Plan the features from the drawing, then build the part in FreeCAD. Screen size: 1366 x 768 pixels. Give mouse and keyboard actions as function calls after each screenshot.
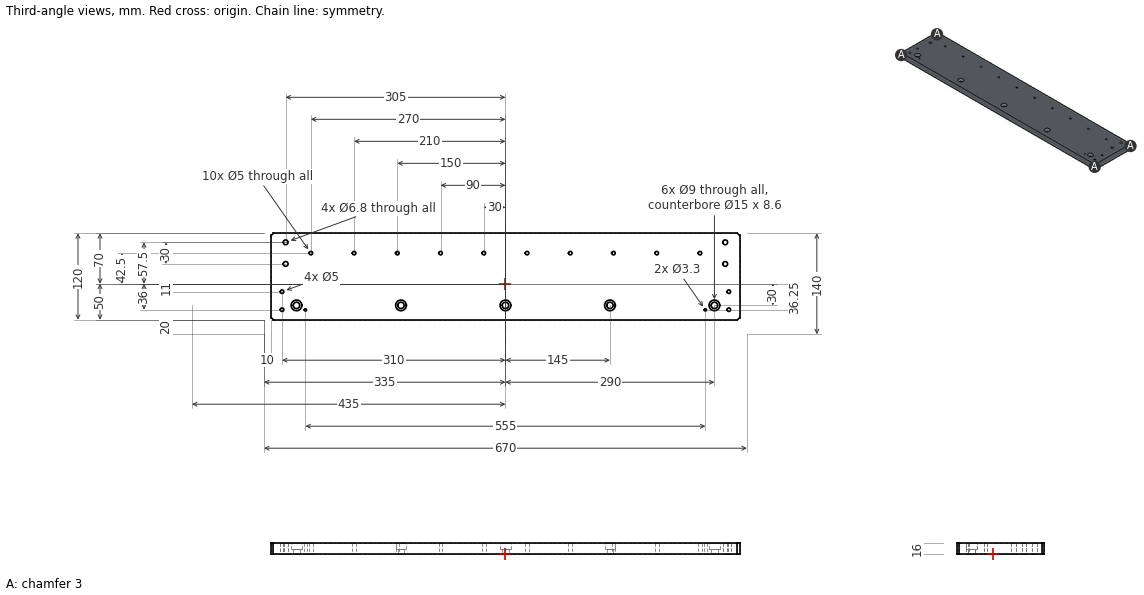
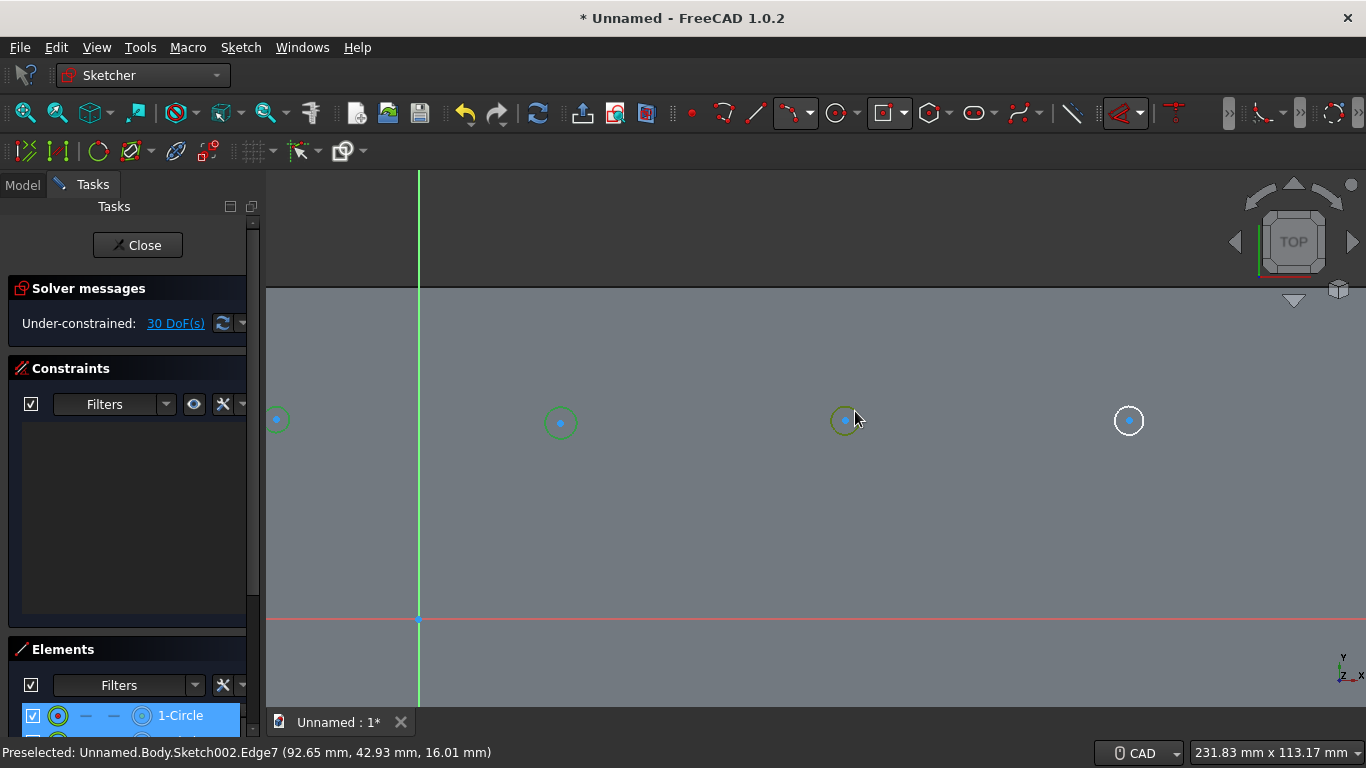
click(1139, 411)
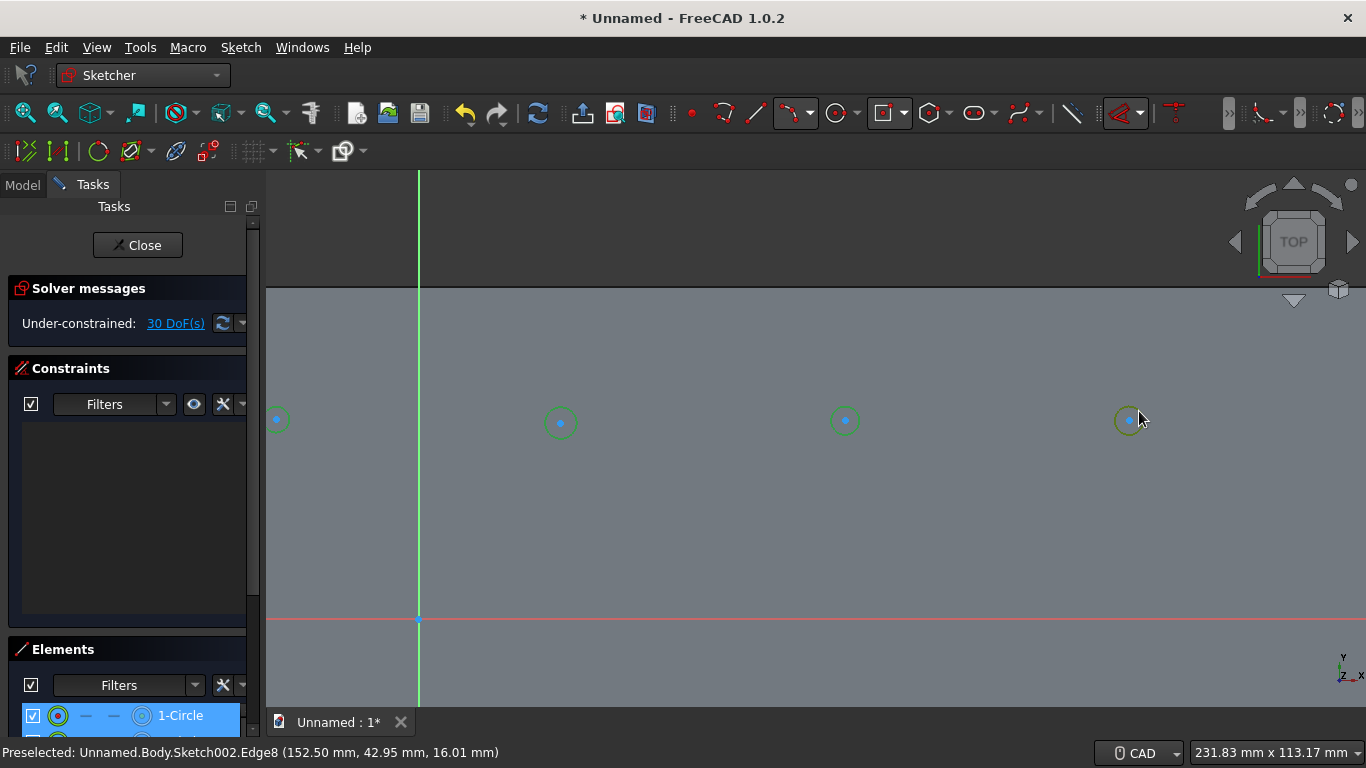
scroll(855, 414, down, 7)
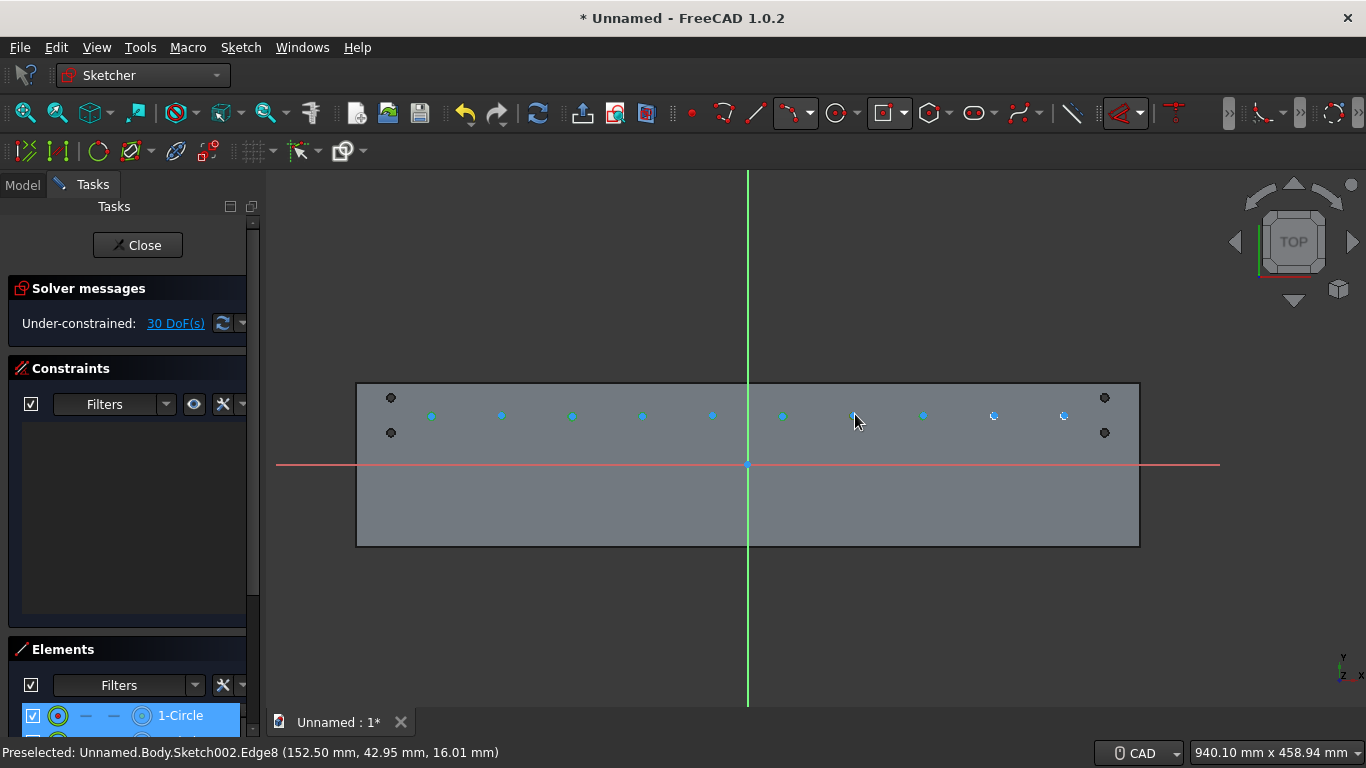
scroll(996, 414, up, 8)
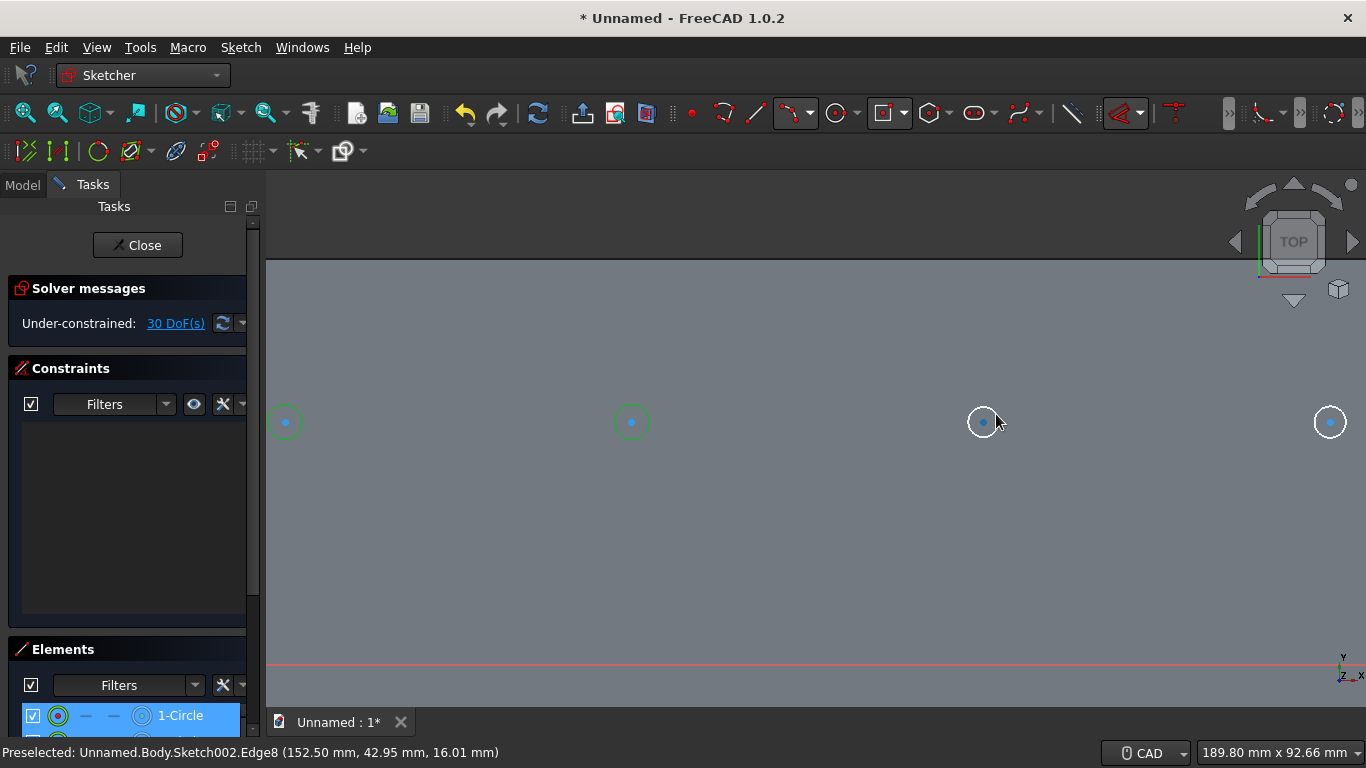
click(994, 411)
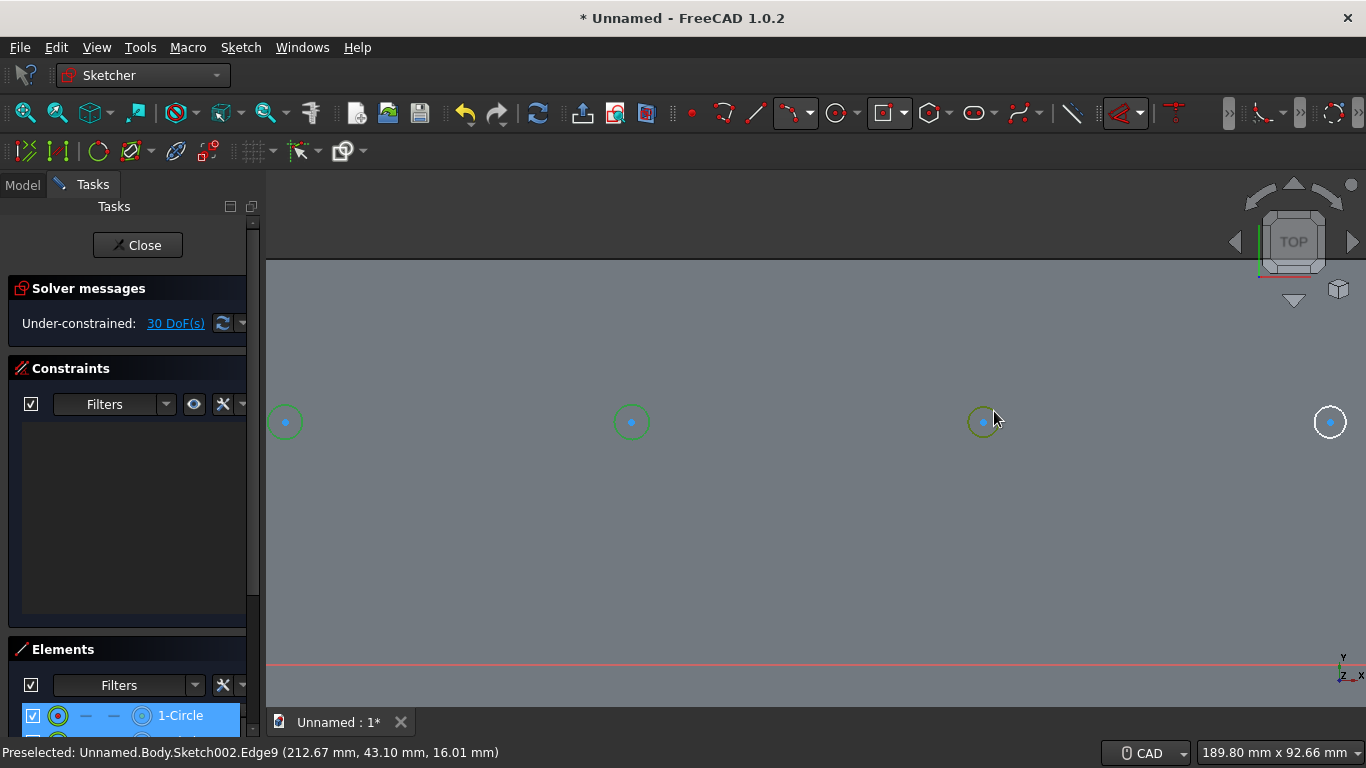
scroll(996, 414, down, 8)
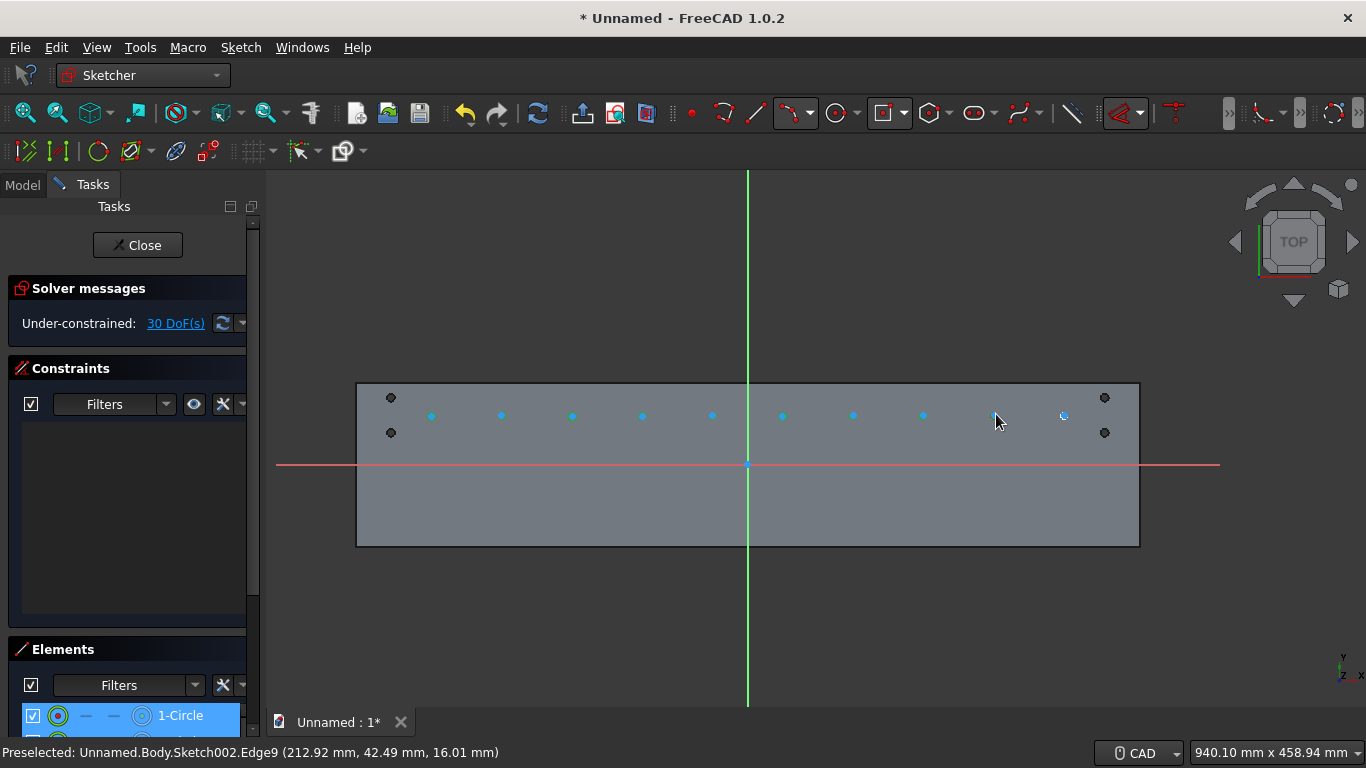
scroll(1066, 414, up, 8)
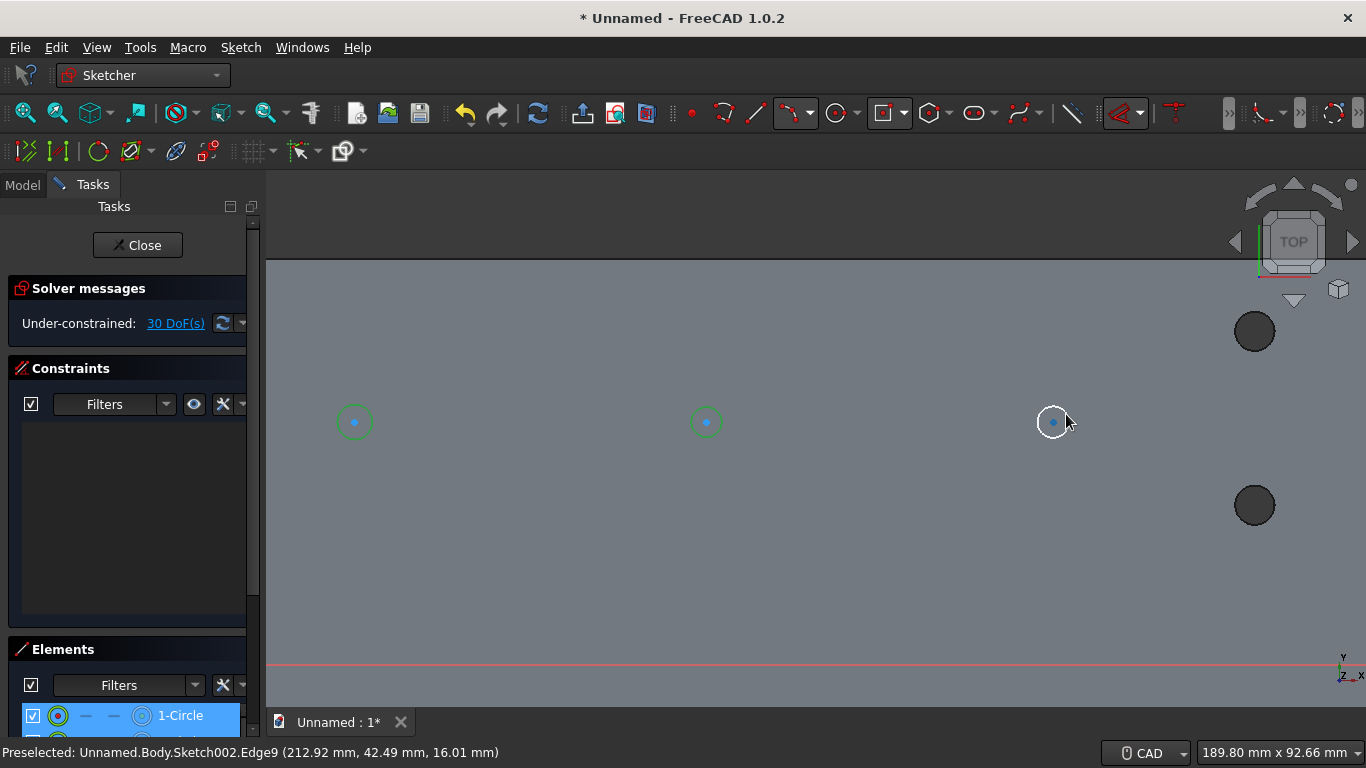
click(1064, 411)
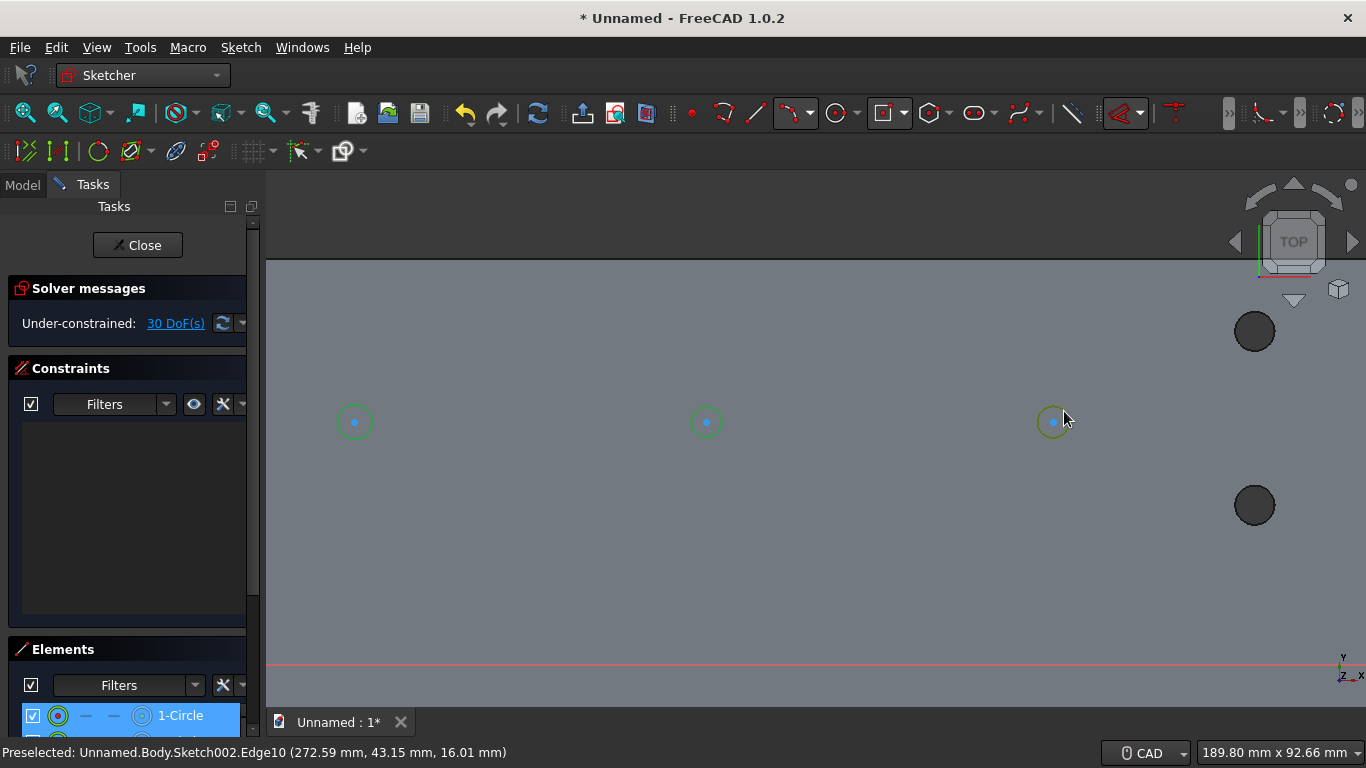
key(e)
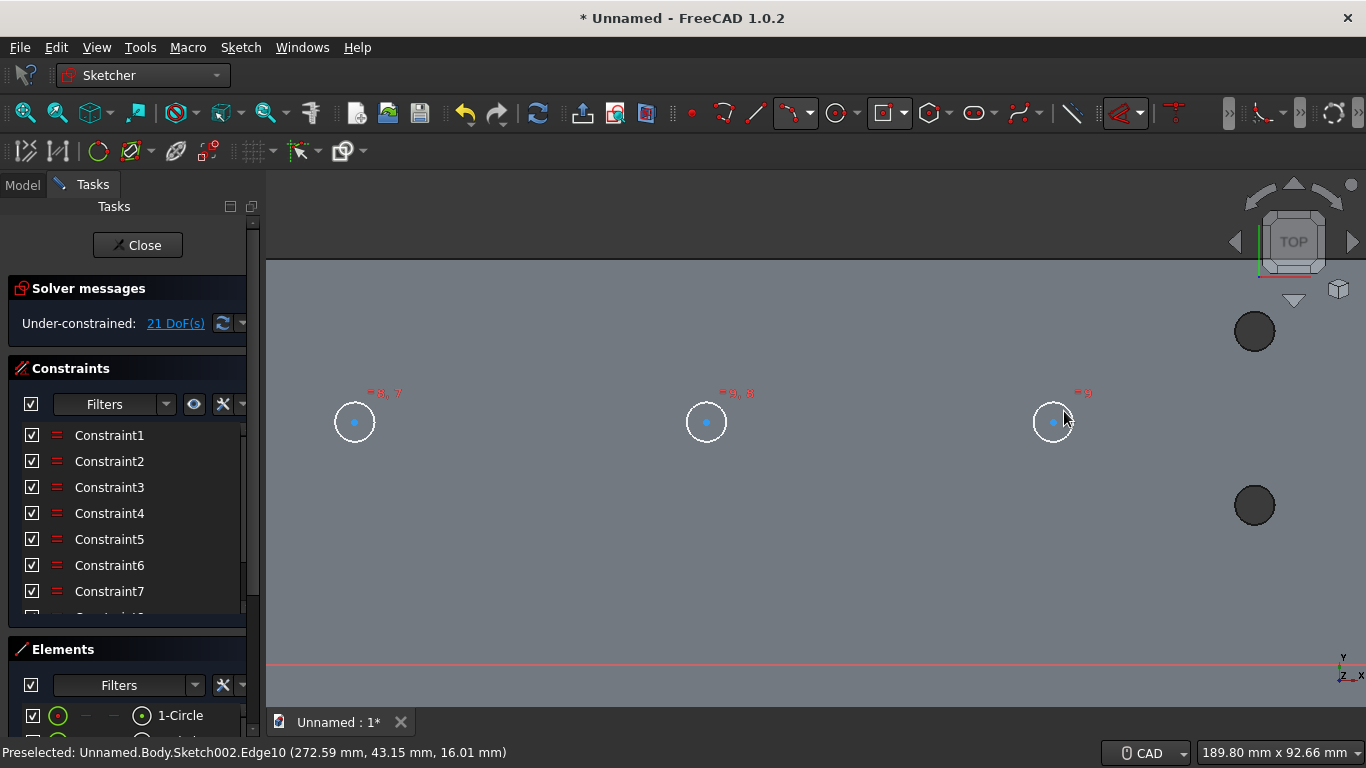
scroll(1066, 414, down, 8)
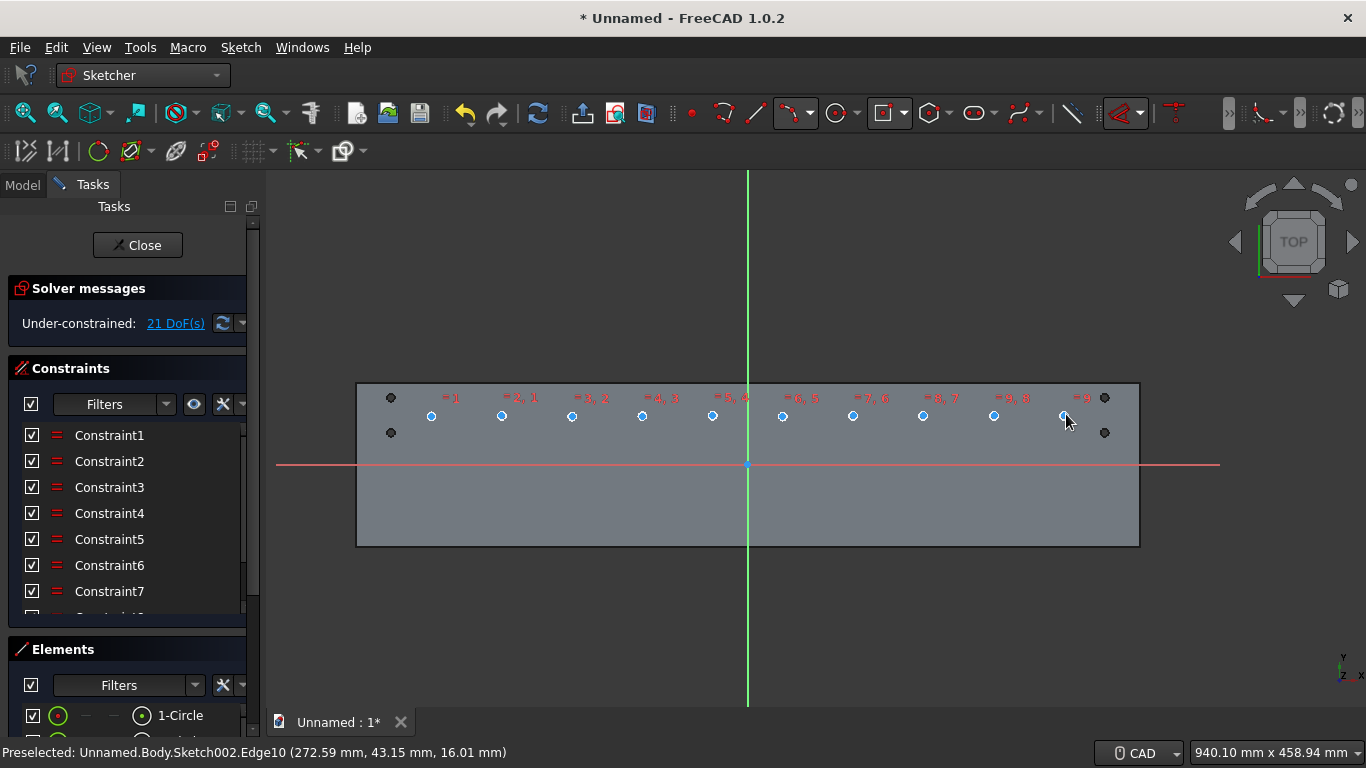
click(713, 416)